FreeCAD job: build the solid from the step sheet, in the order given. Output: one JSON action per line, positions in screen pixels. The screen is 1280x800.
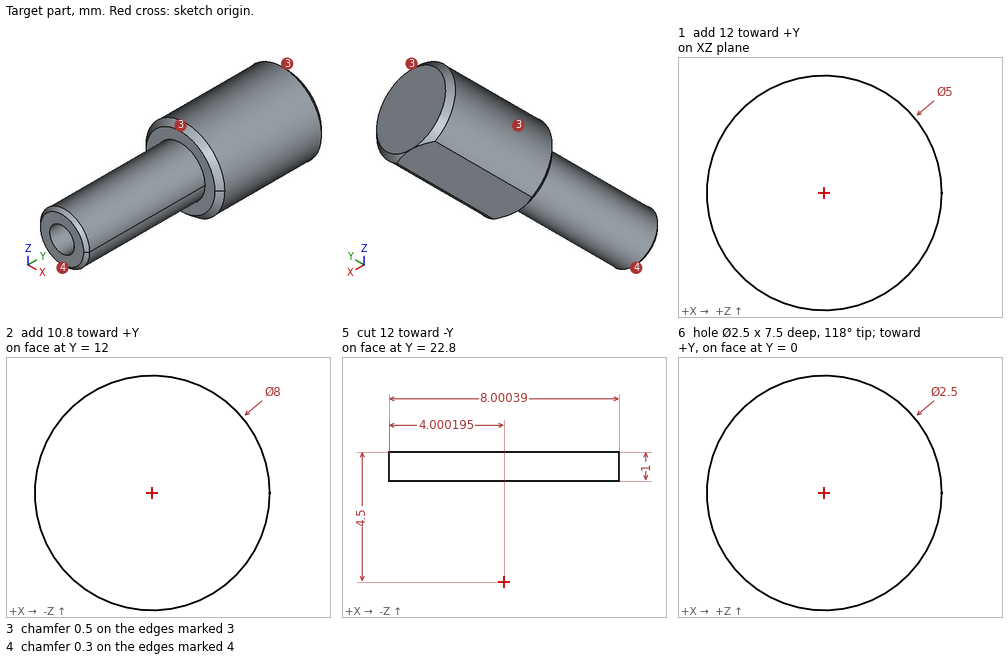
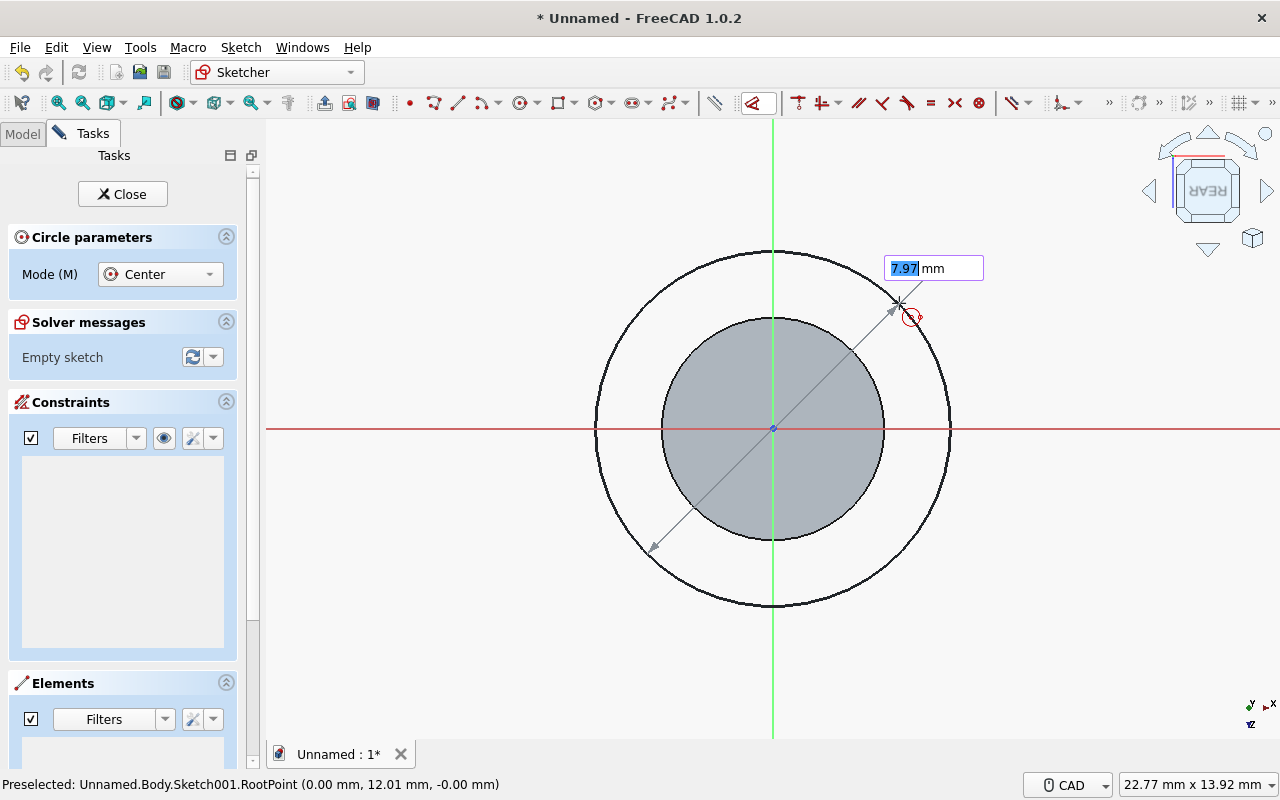
{"action": "type", "text": "8"}
{"action": "key", "text": "Return"}
{"action": "key", "text": "Escape"}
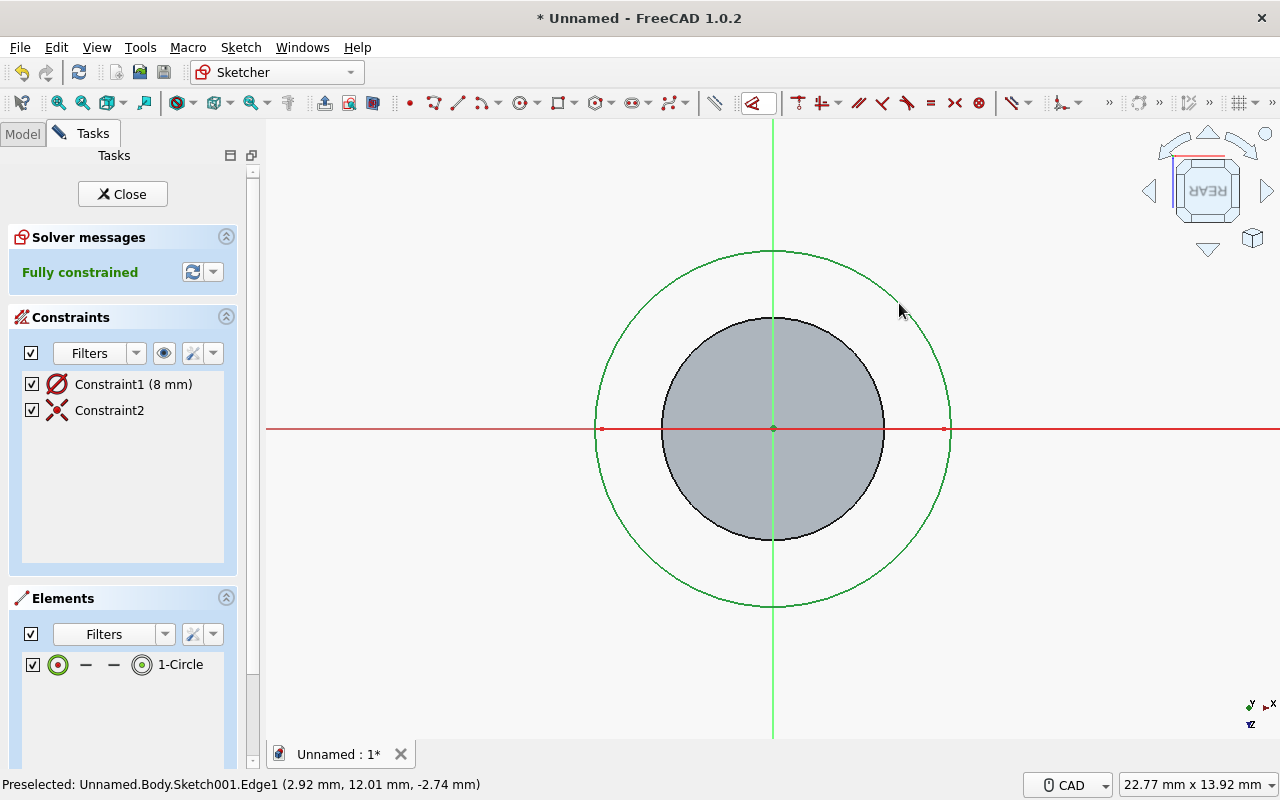
{"action": "left_click", "coordinate": [123, 194]}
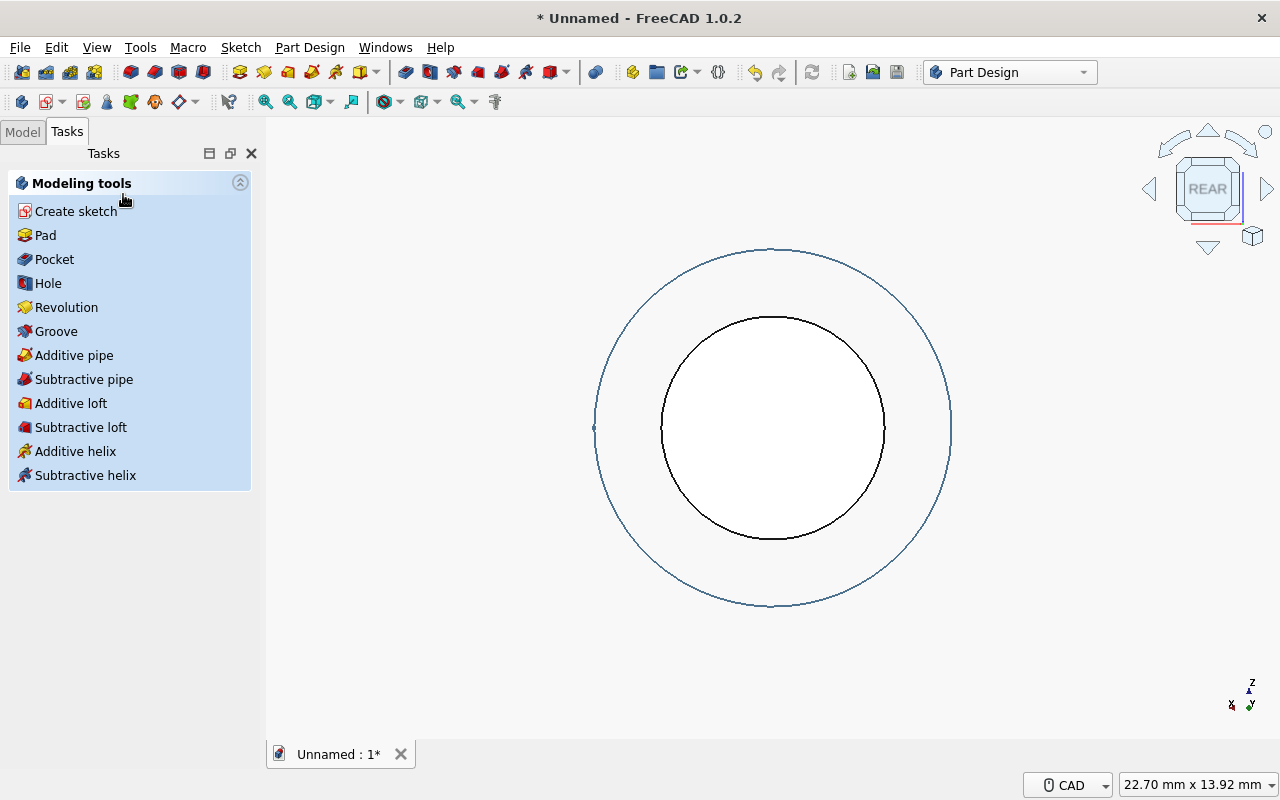
{"action": "left_click", "coordinate": [240, 72]}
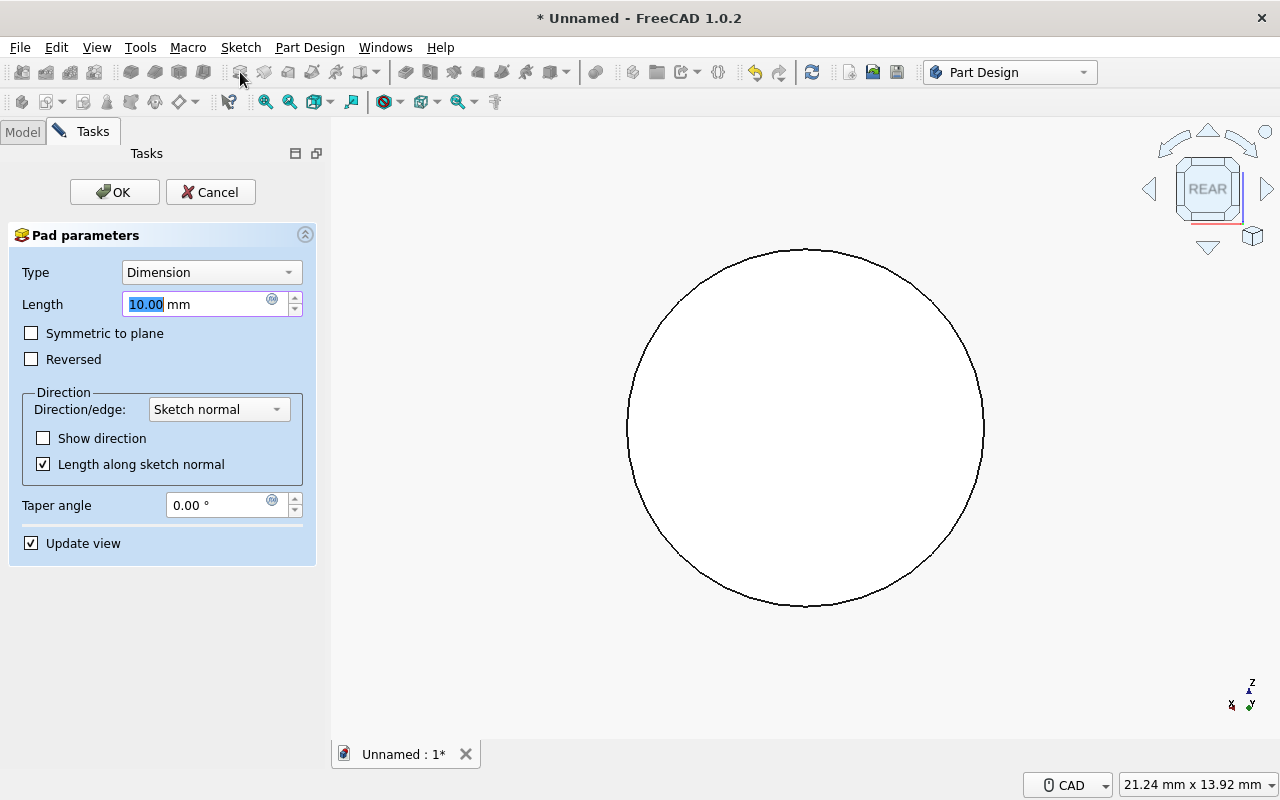
{"action": "type", "text": "10.8"}
{"action": "key", "text": "Tab"}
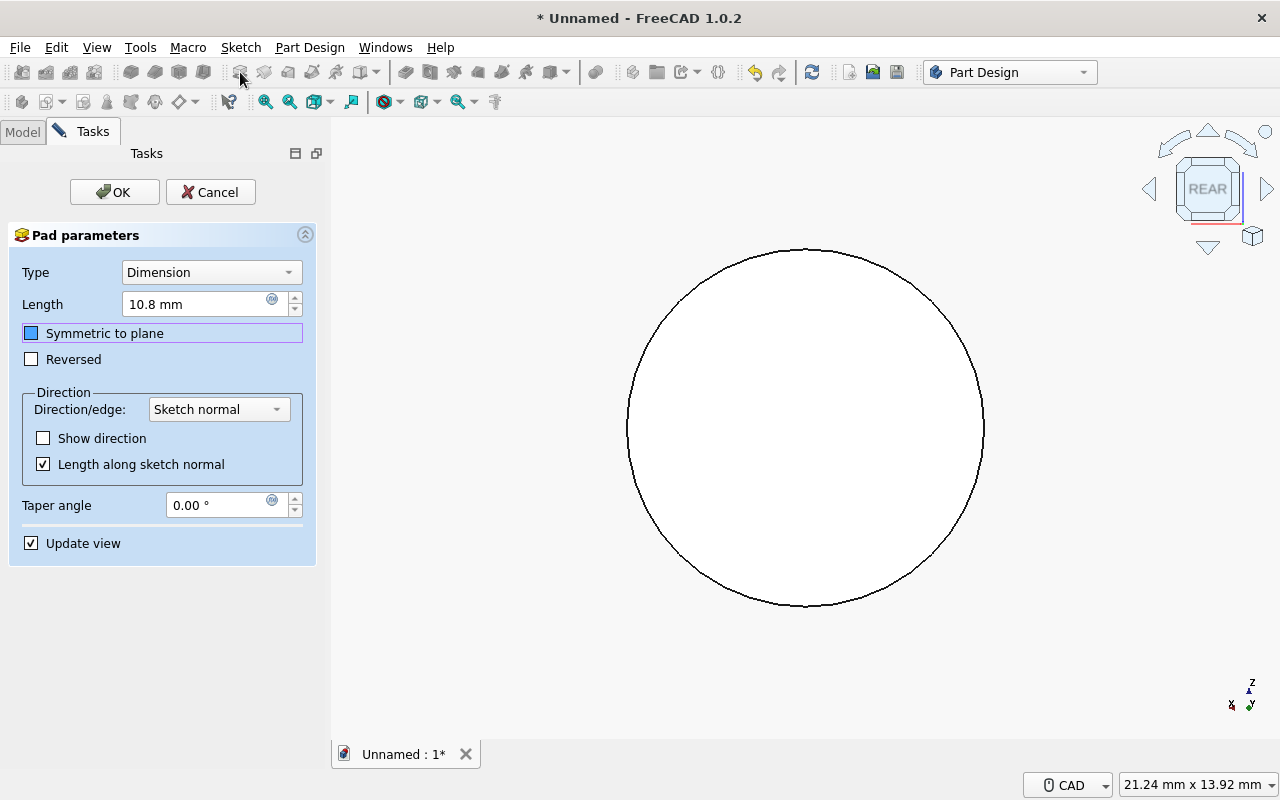
{"action": "left_click", "coordinate": [115, 192]}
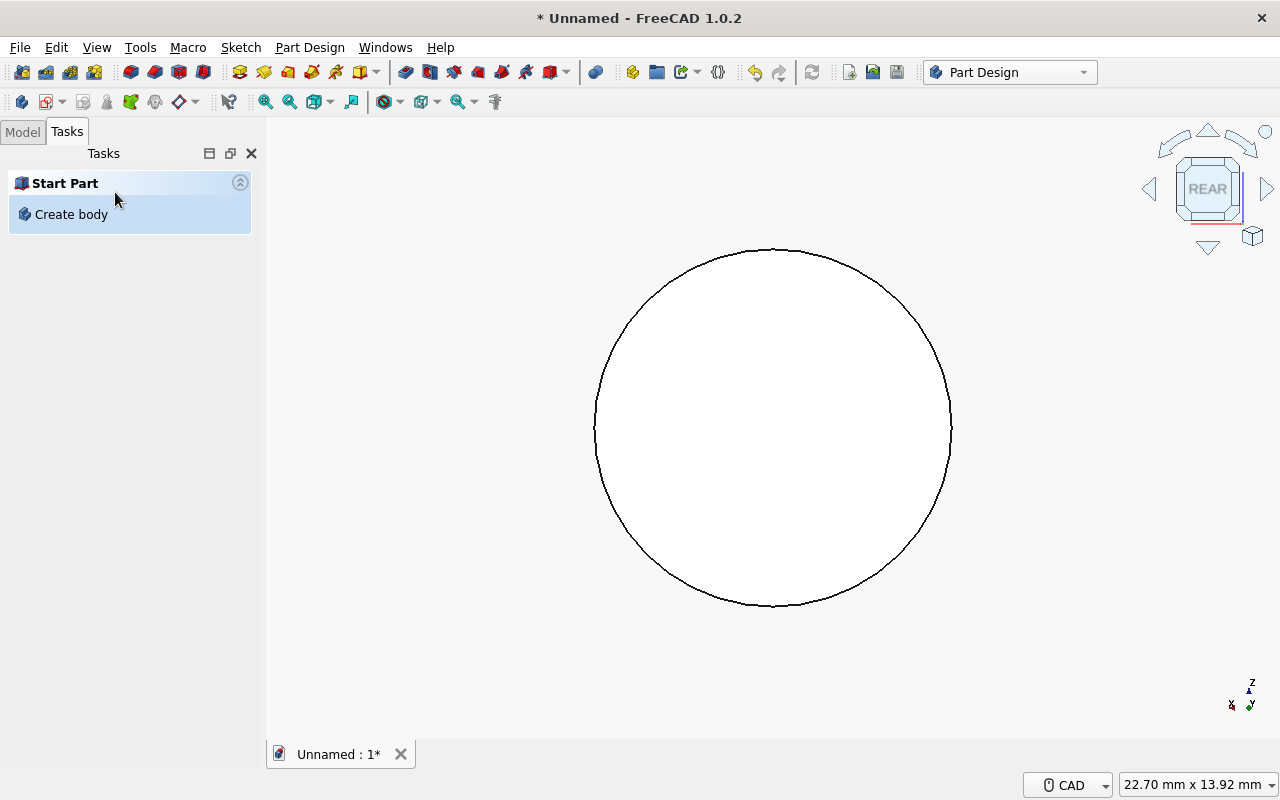
{"action": "left_click", "coordinate": [952, 427]}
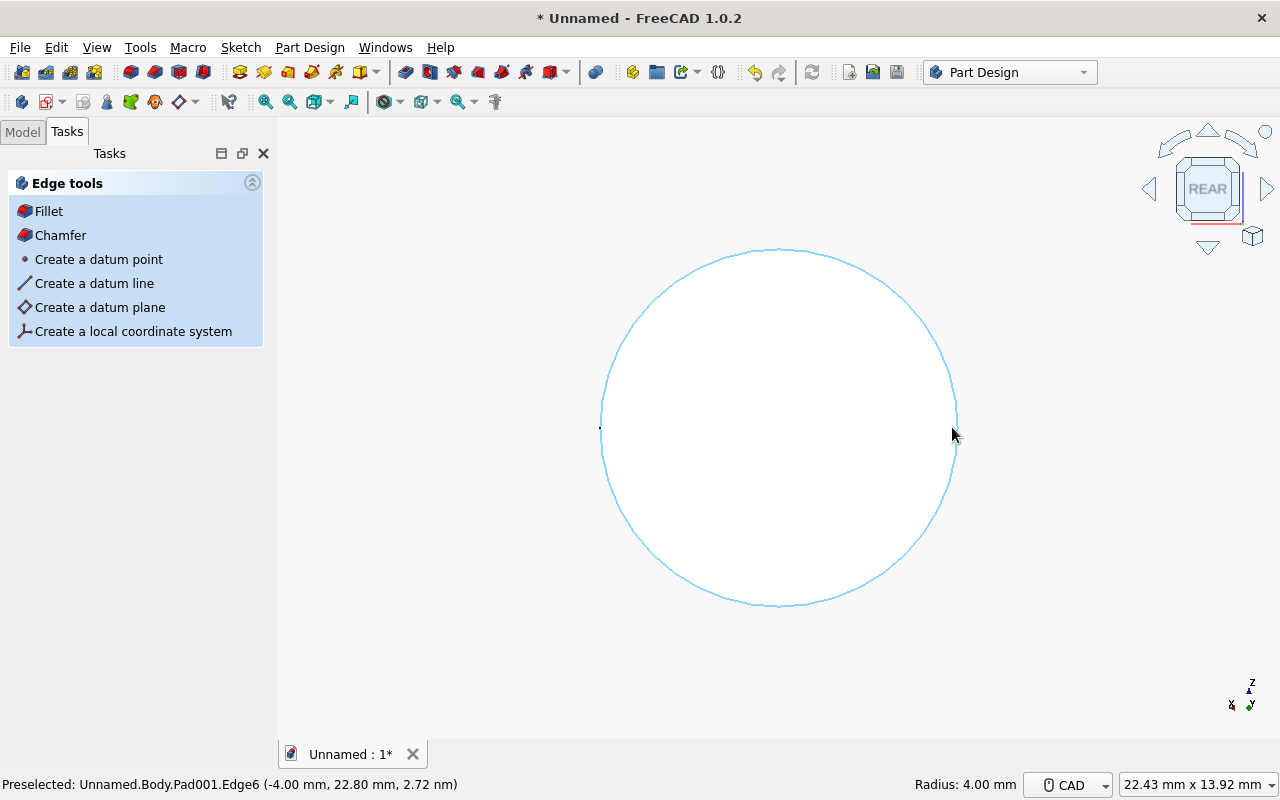
{"action": "key", "text": "0"}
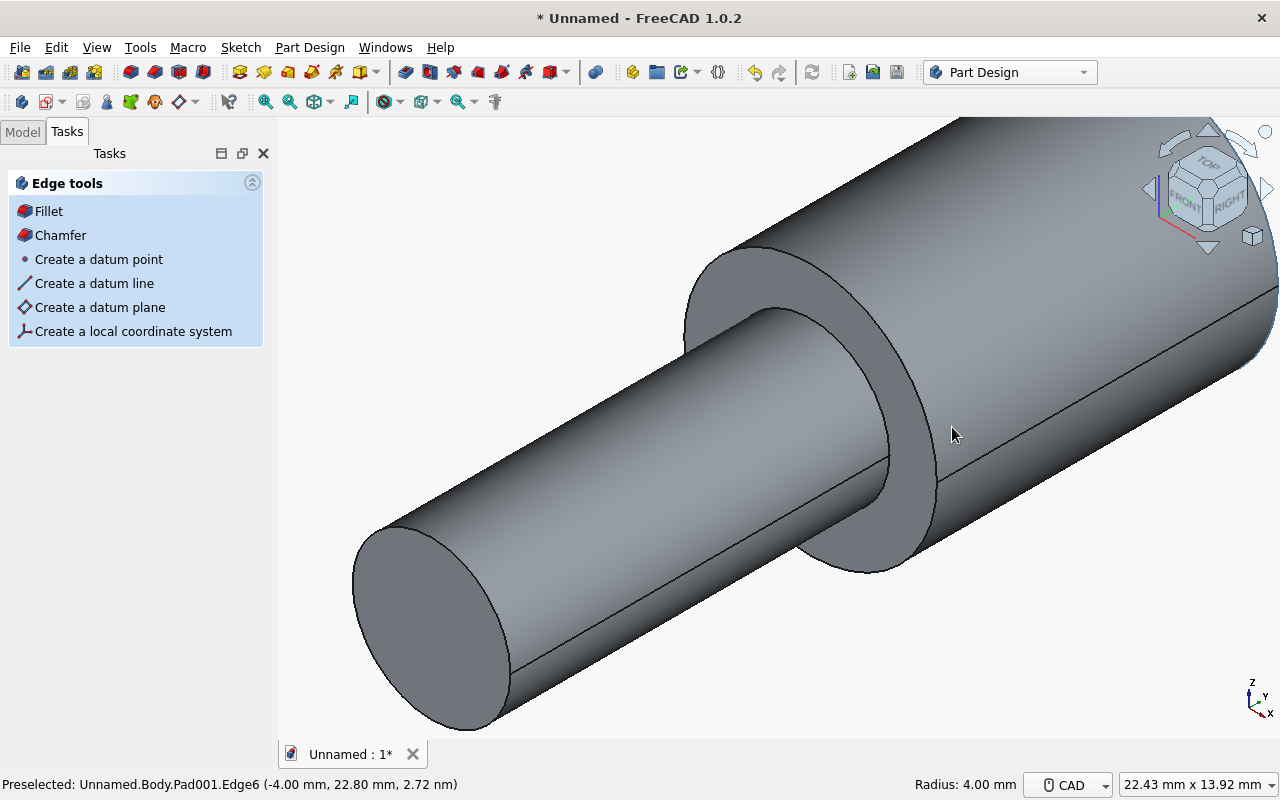
{"action": "left_click", "coordinate": [266, 102]}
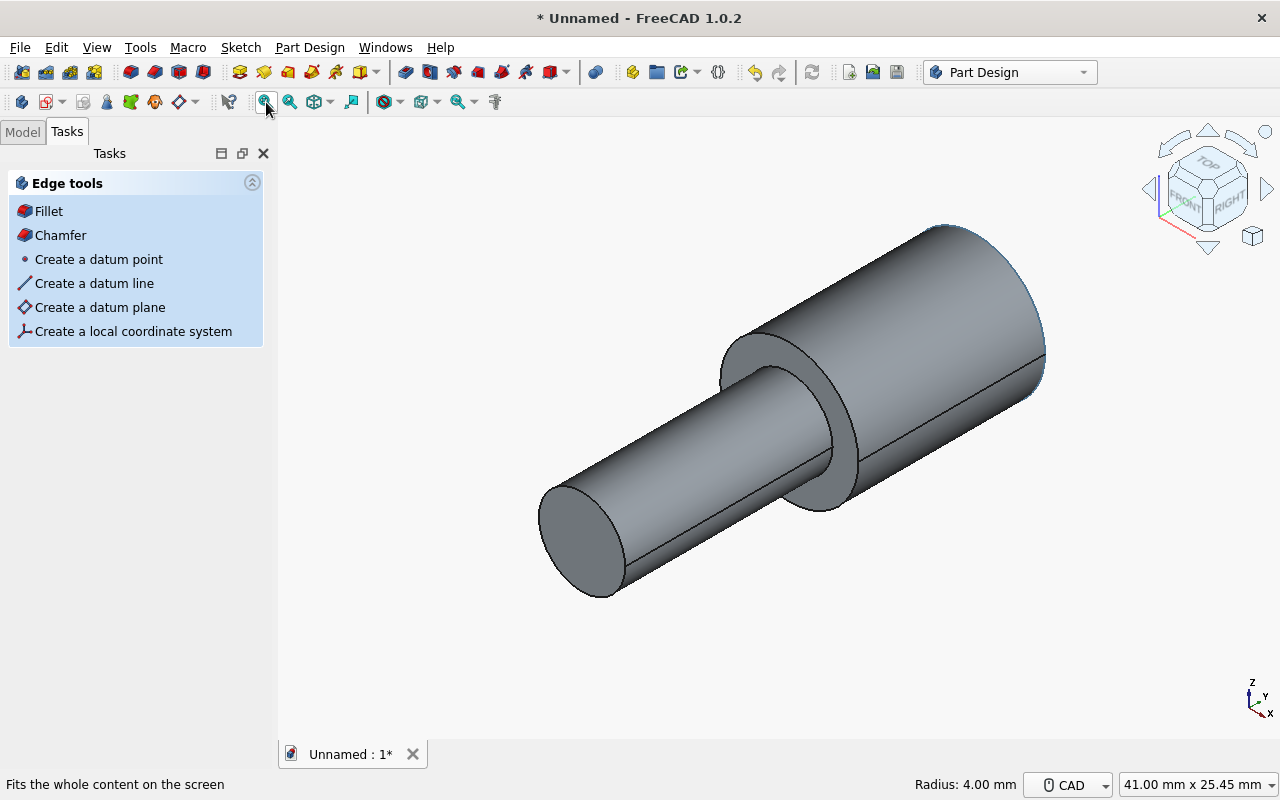
{"action": "left_click", "coordinate": [733, 342], "text": "ctrl"}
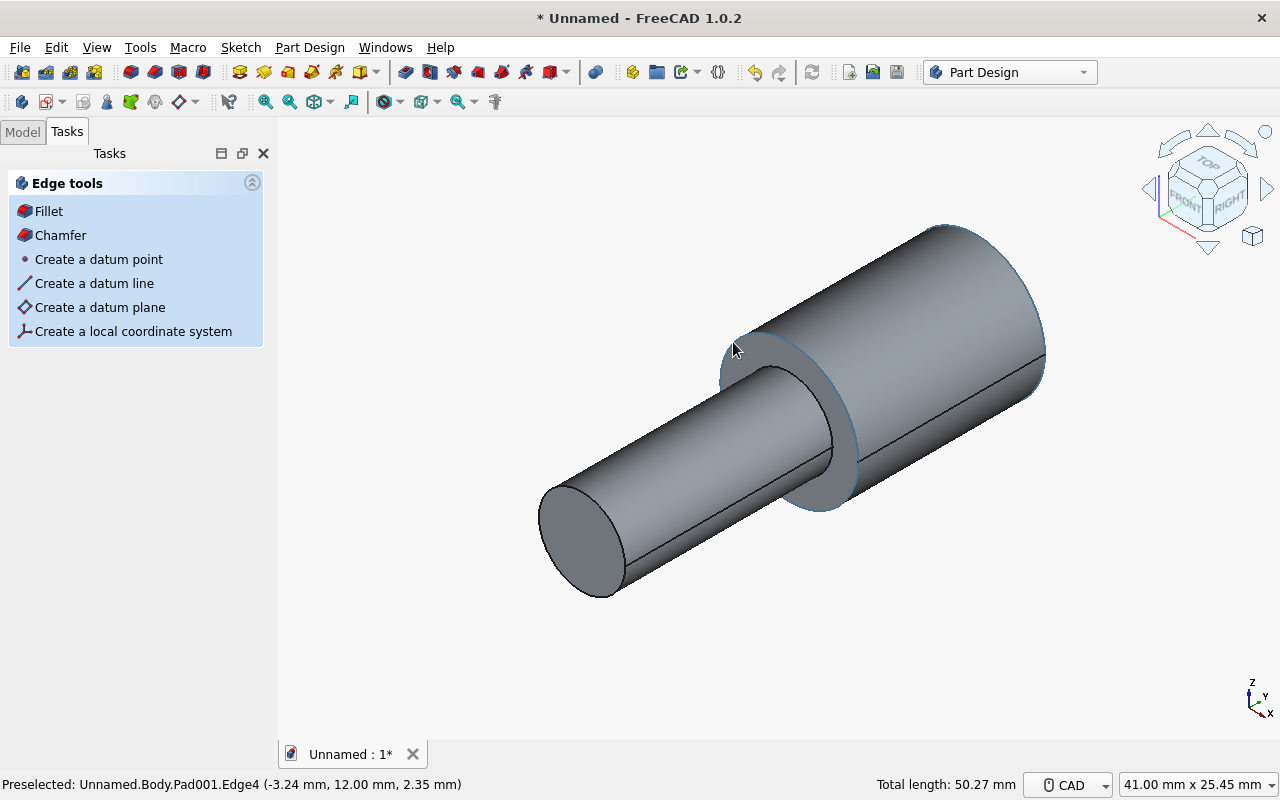
{"action": "left_click", "coordinate": [156, 72]}